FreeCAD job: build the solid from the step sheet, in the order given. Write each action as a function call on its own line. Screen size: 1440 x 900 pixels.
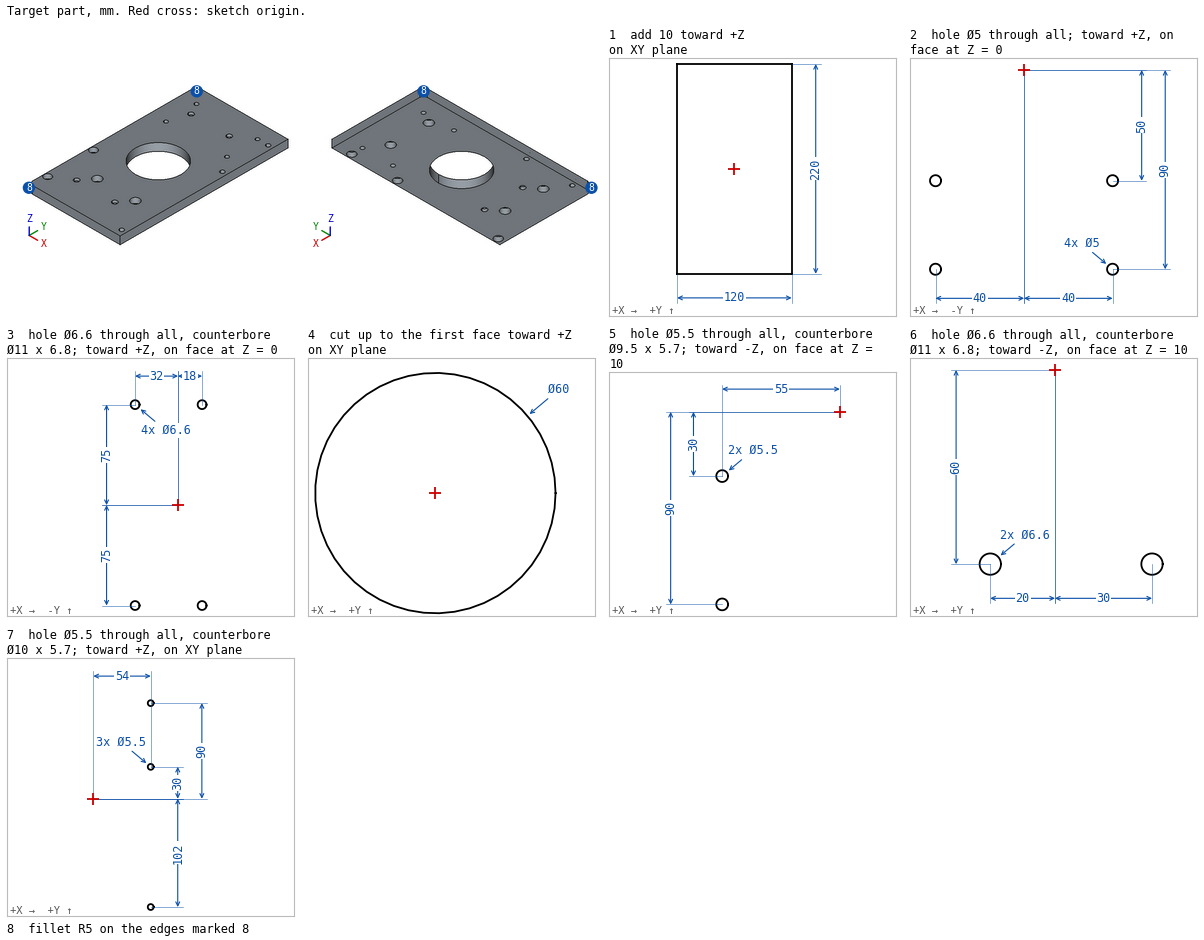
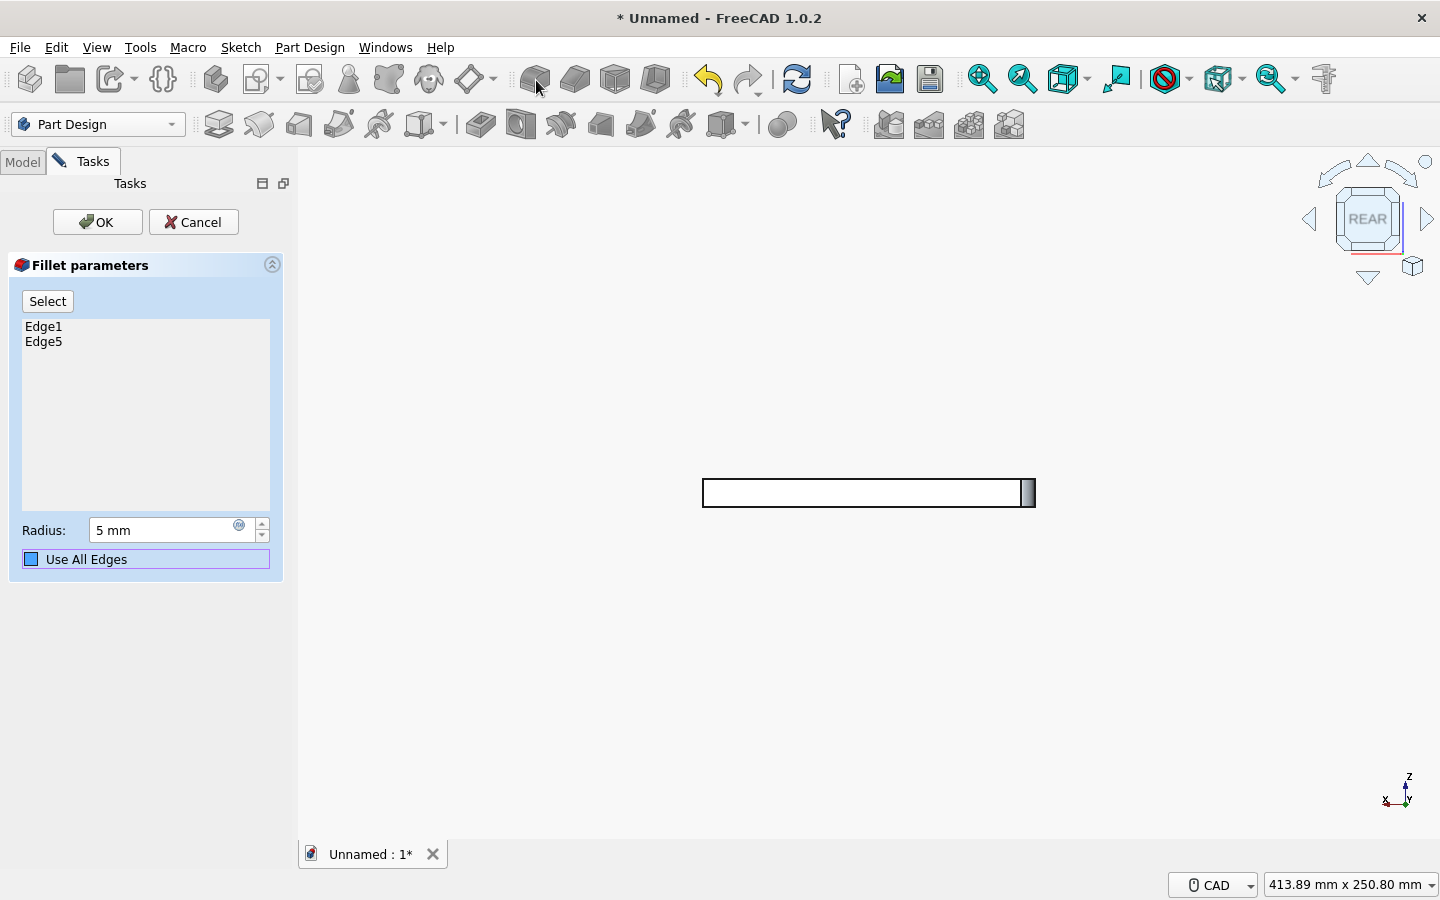
click(98, 222)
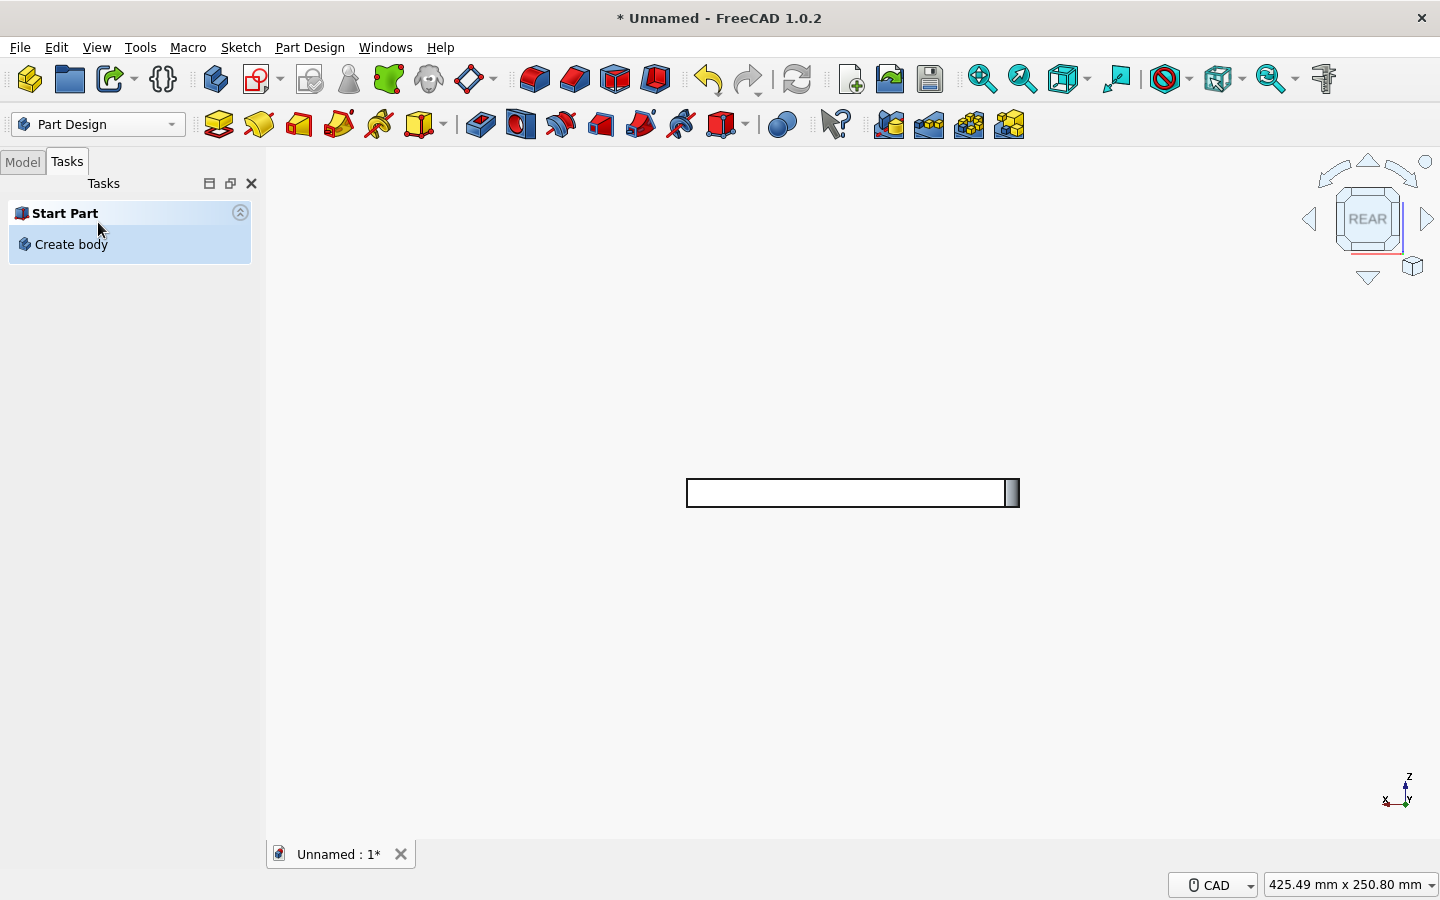
key(0)